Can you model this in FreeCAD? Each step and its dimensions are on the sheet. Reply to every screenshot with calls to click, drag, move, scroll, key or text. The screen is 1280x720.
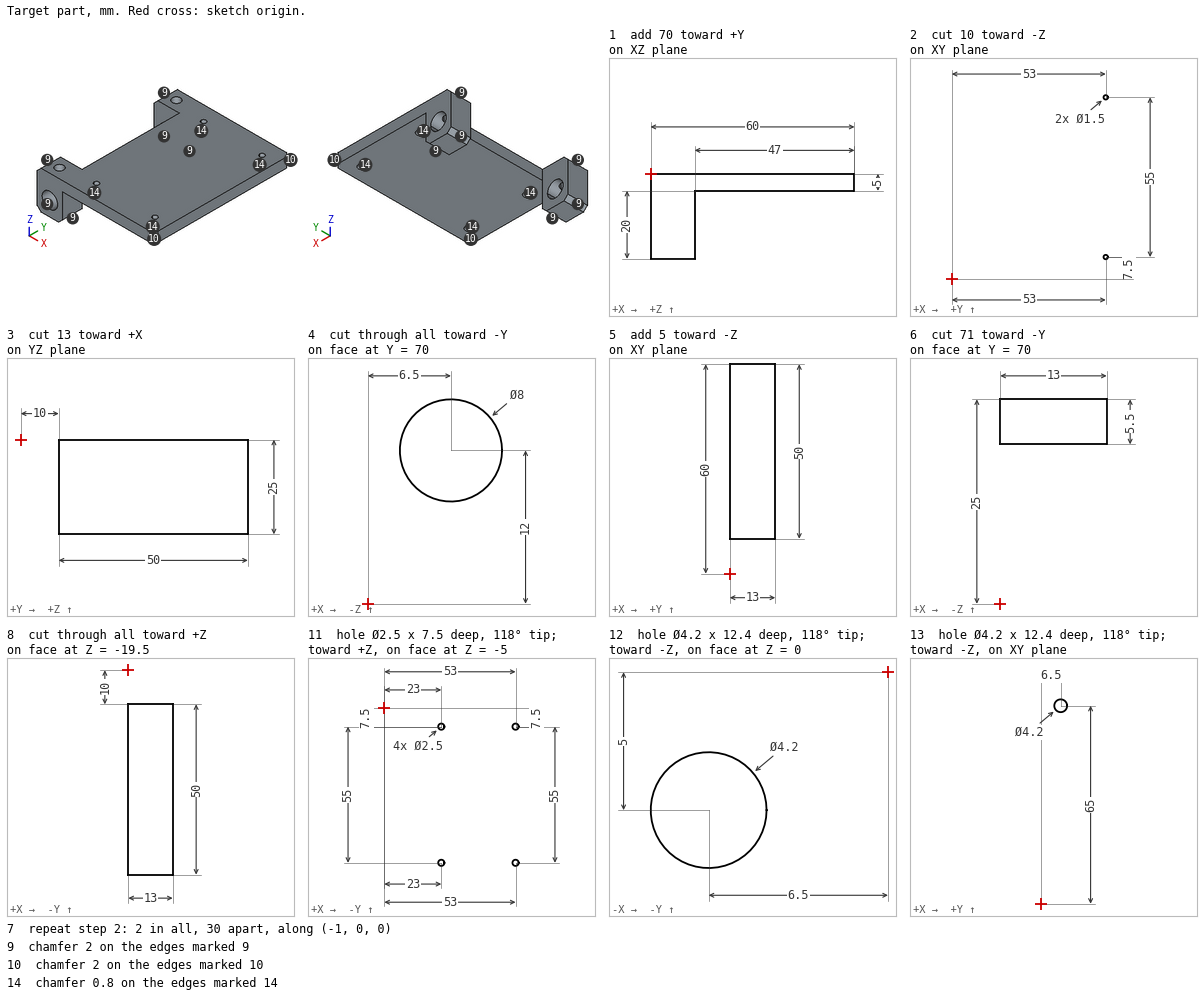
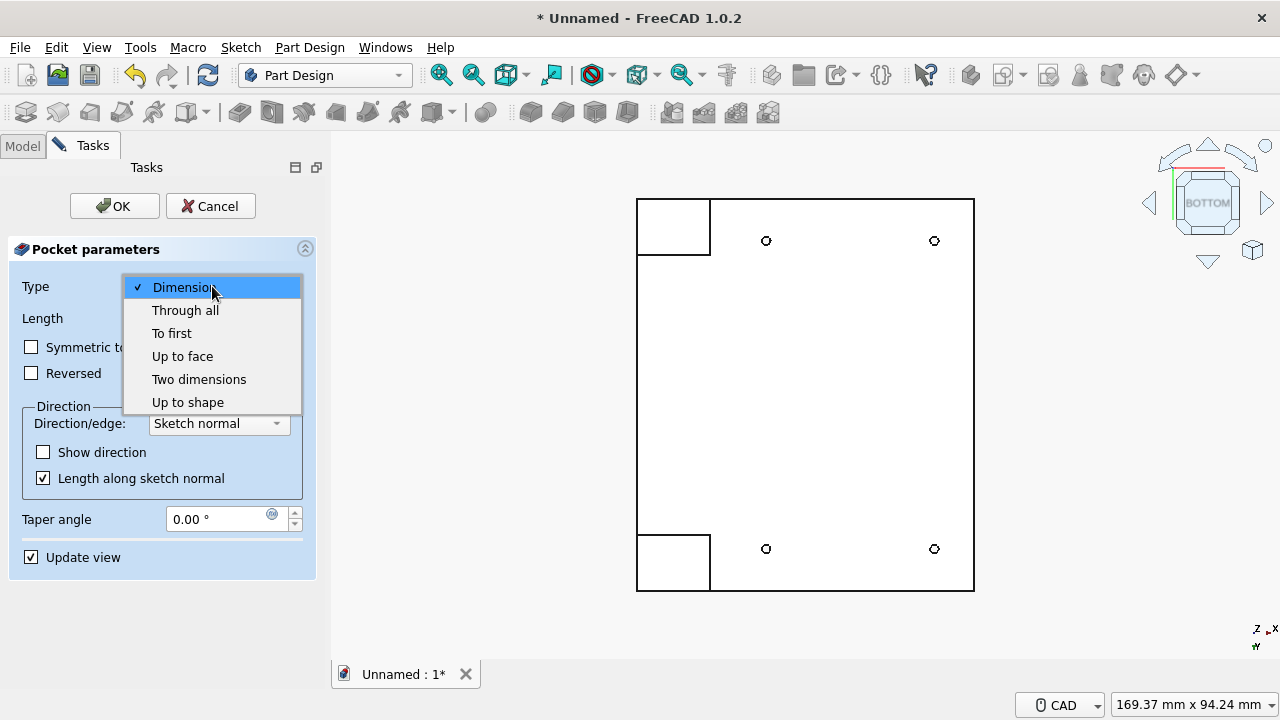
click(212, 310)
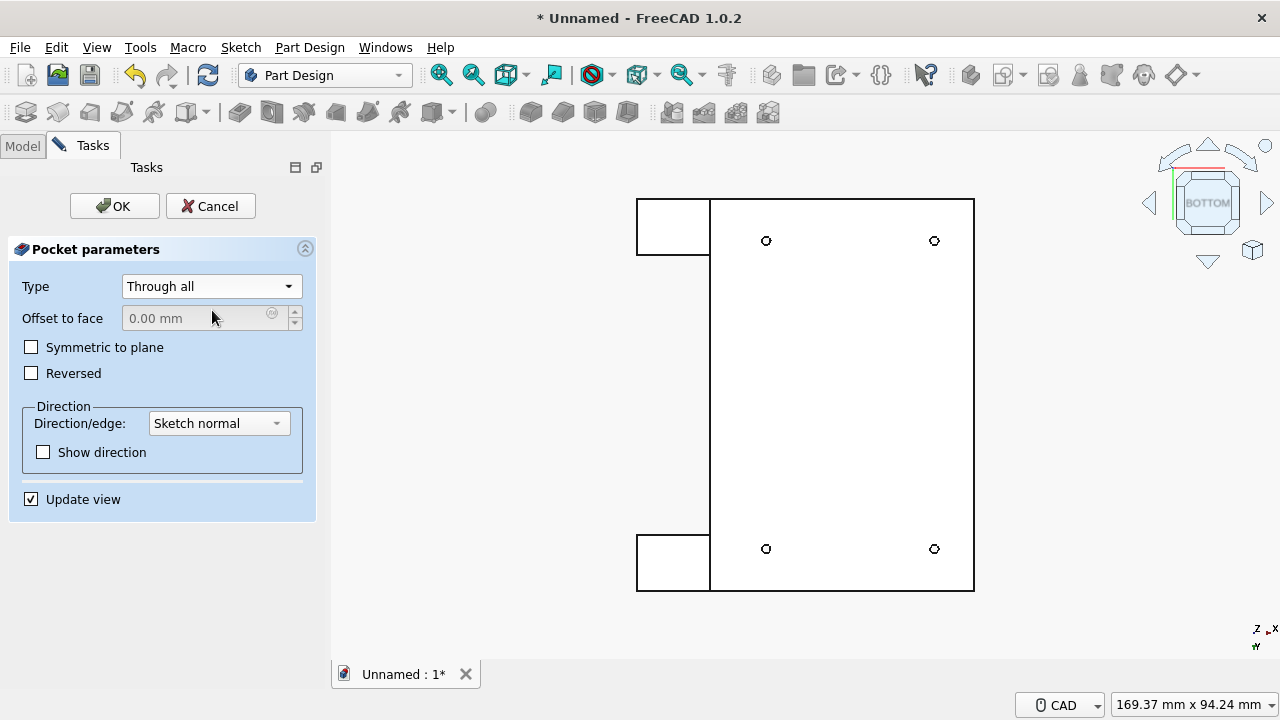
click(115, 206)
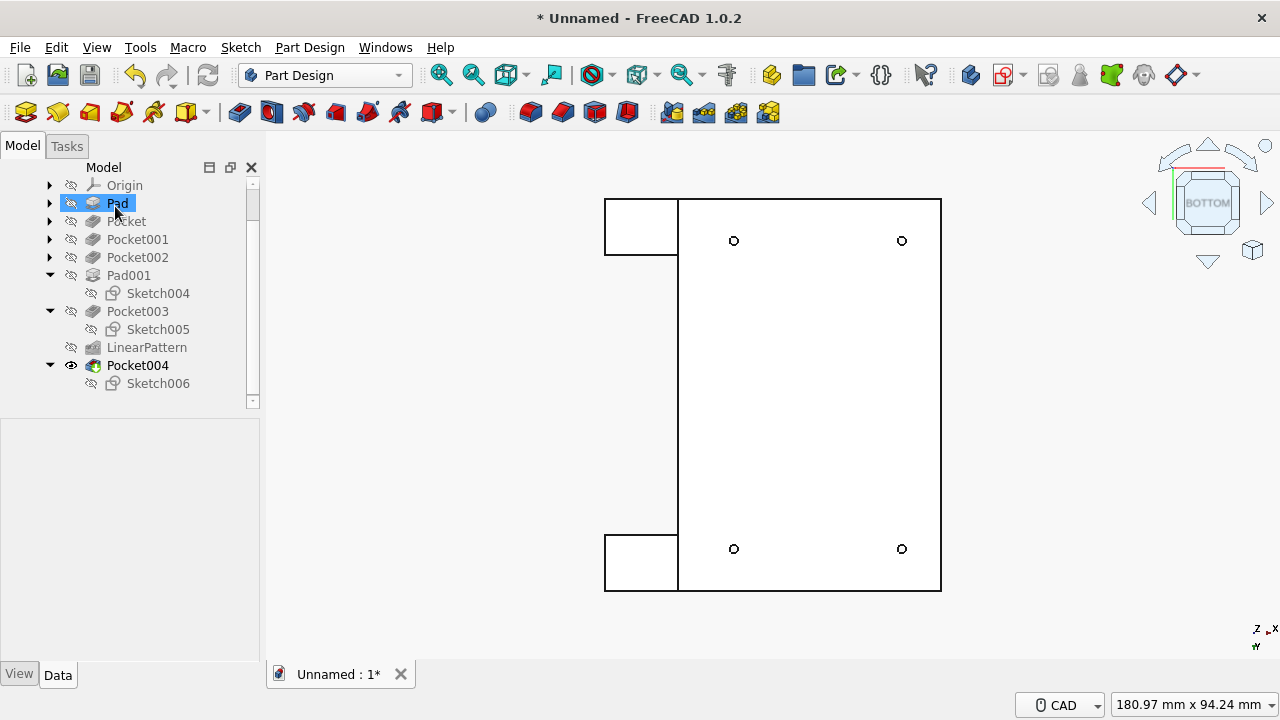
click(605, 226)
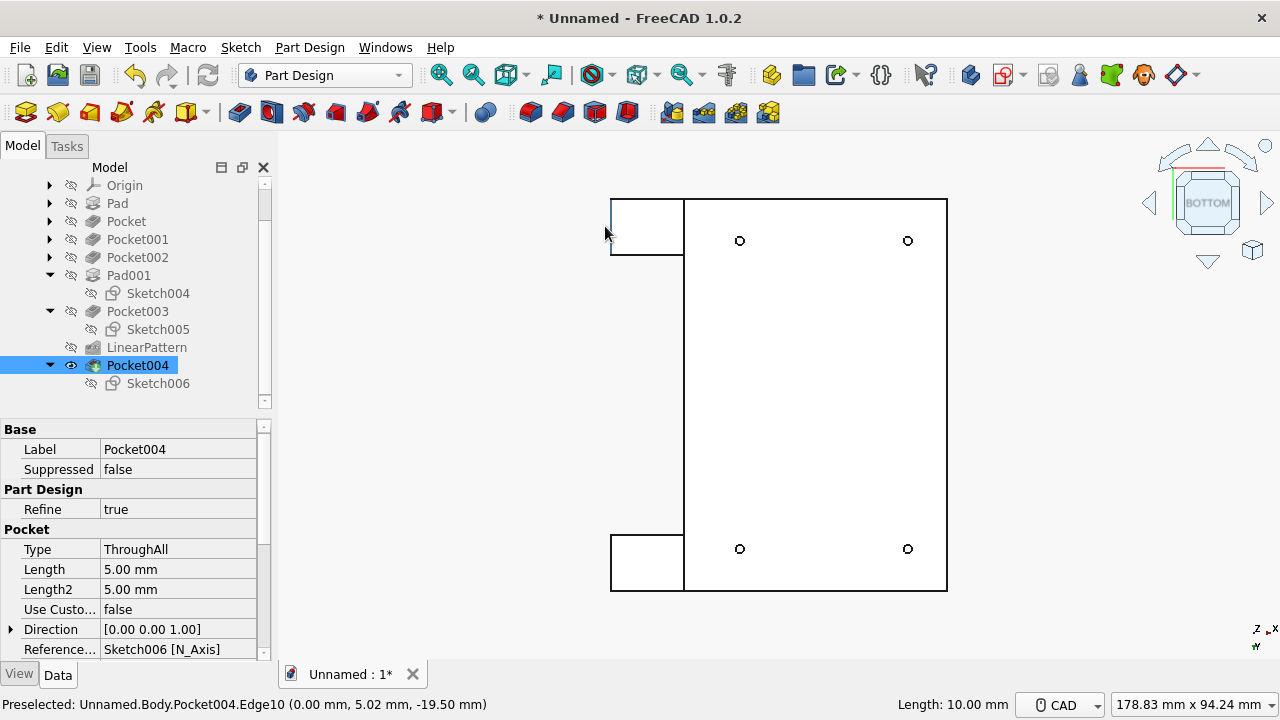
click(611, 562, ctrl)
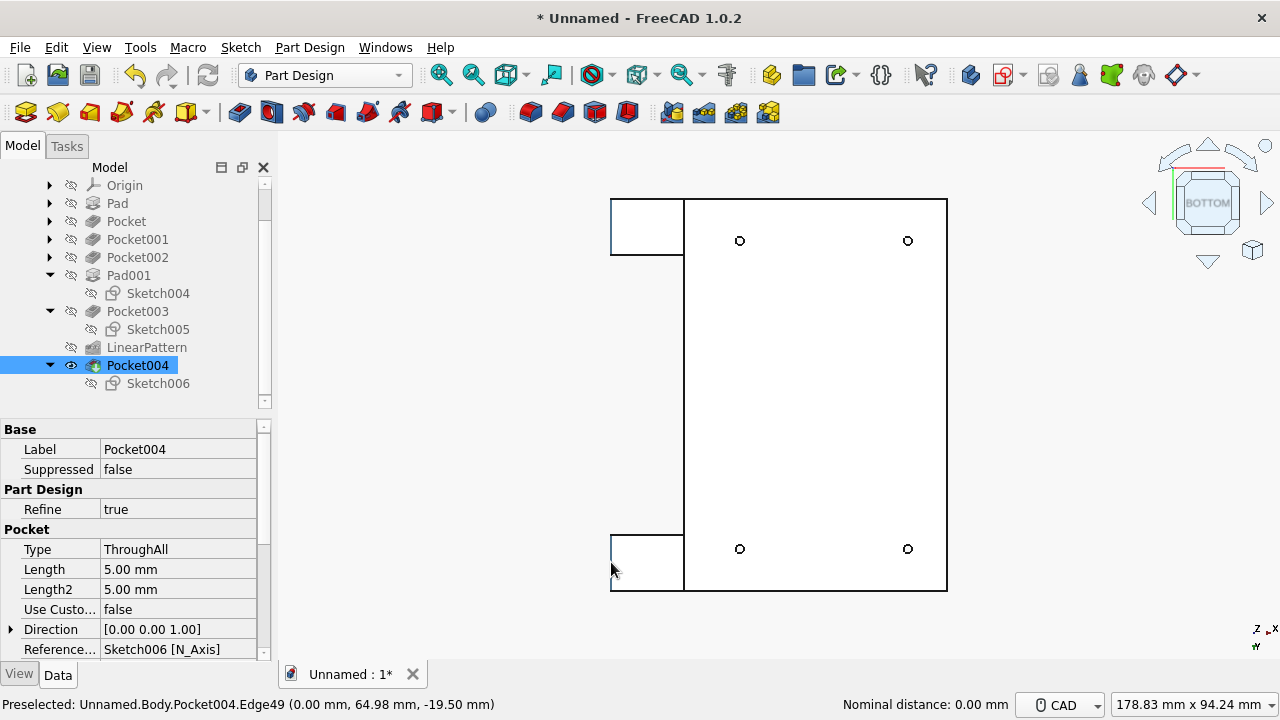
click(684, 226, ctrl)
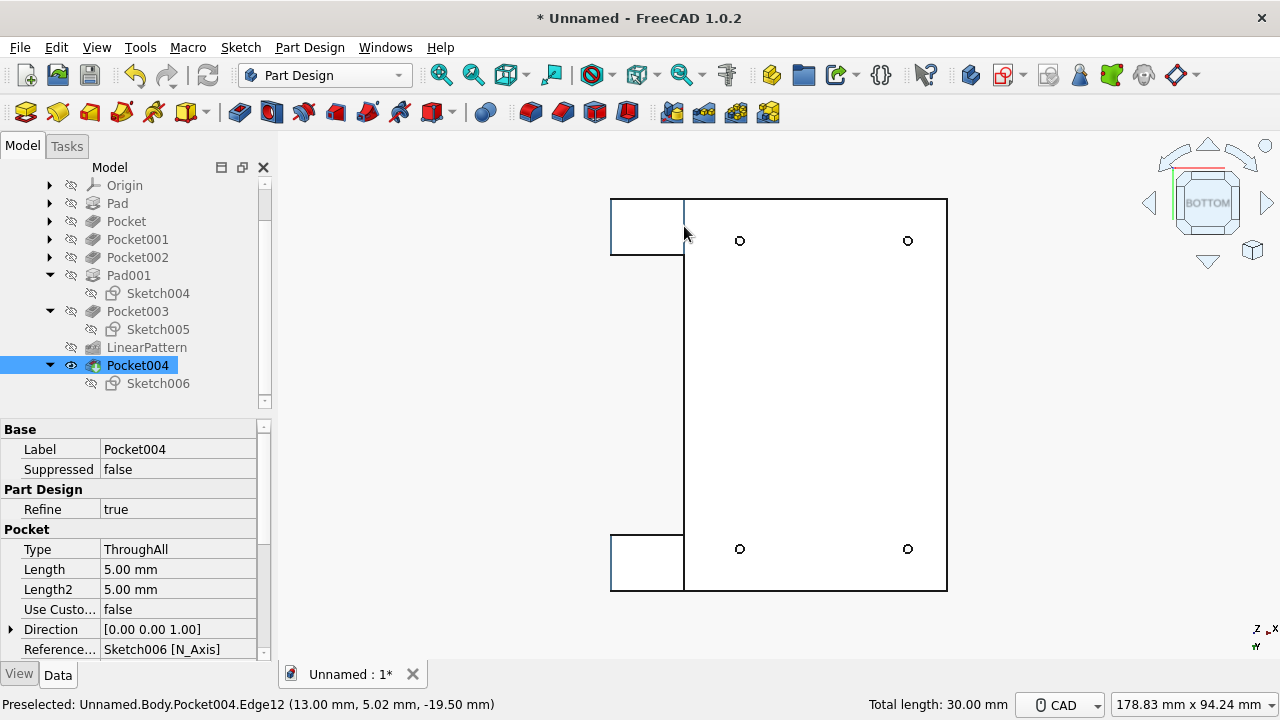
click(684, 562, ctrl)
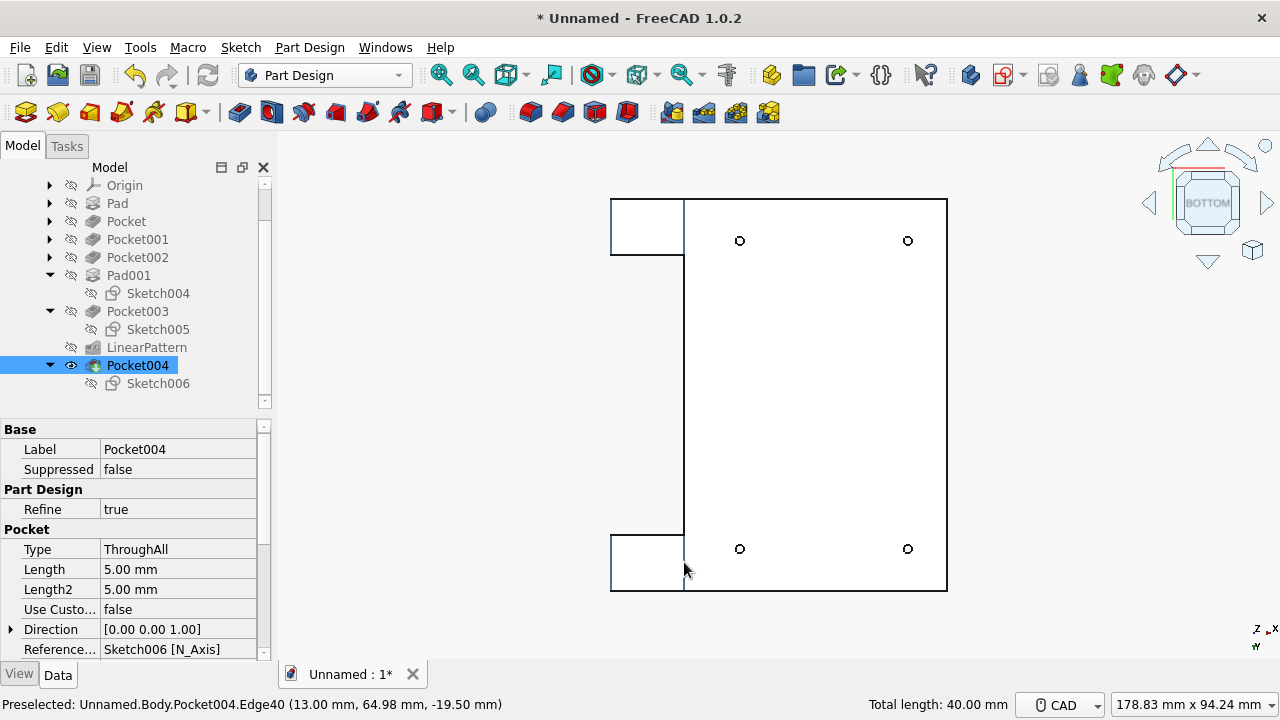
key(0)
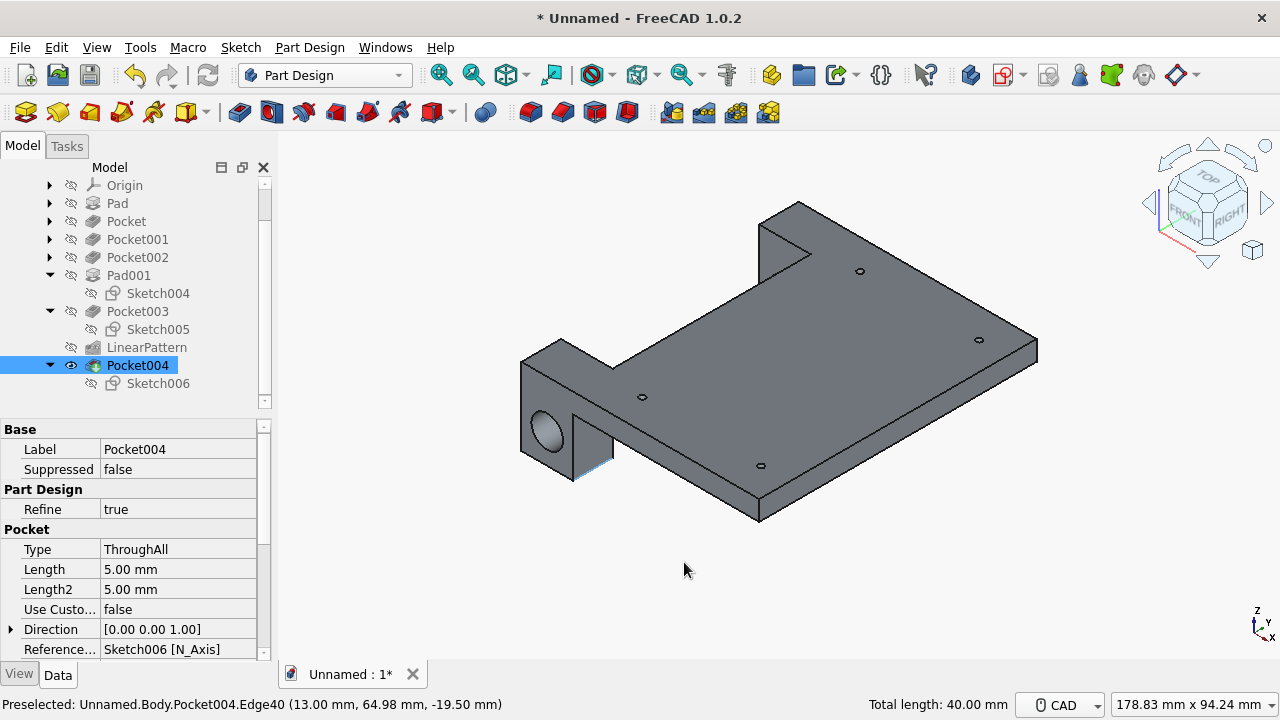
key(2)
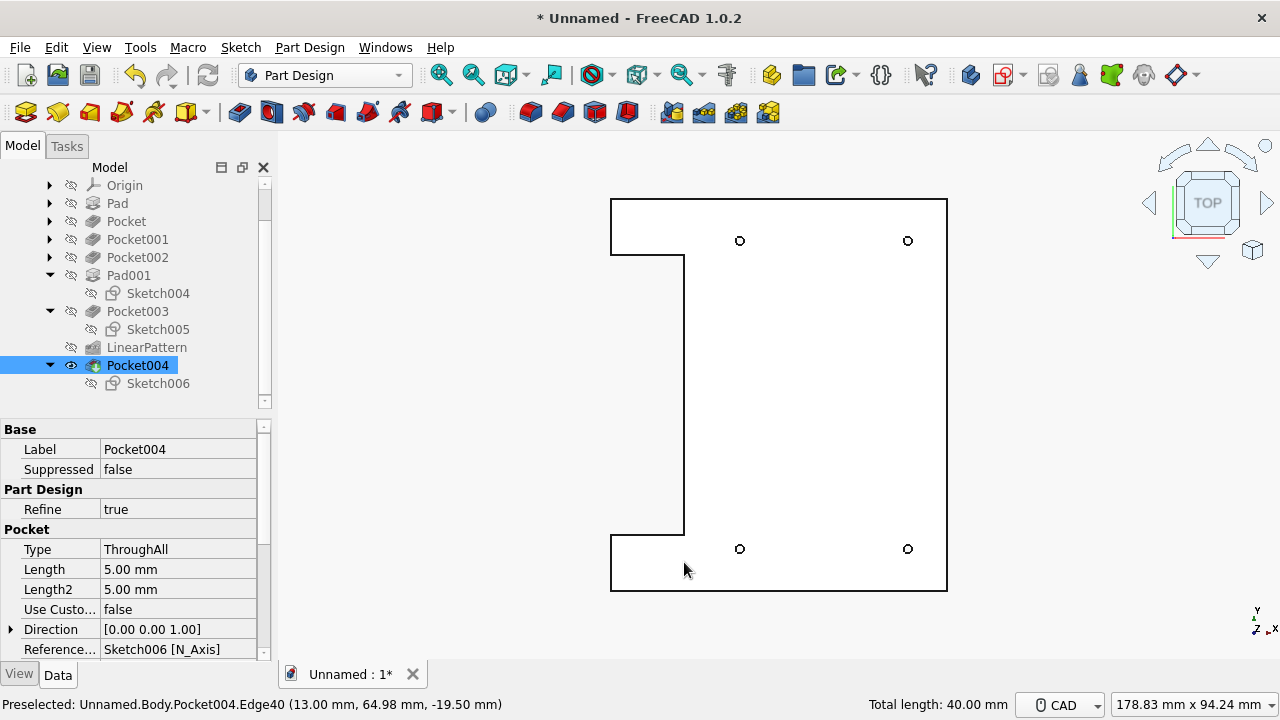
key(1)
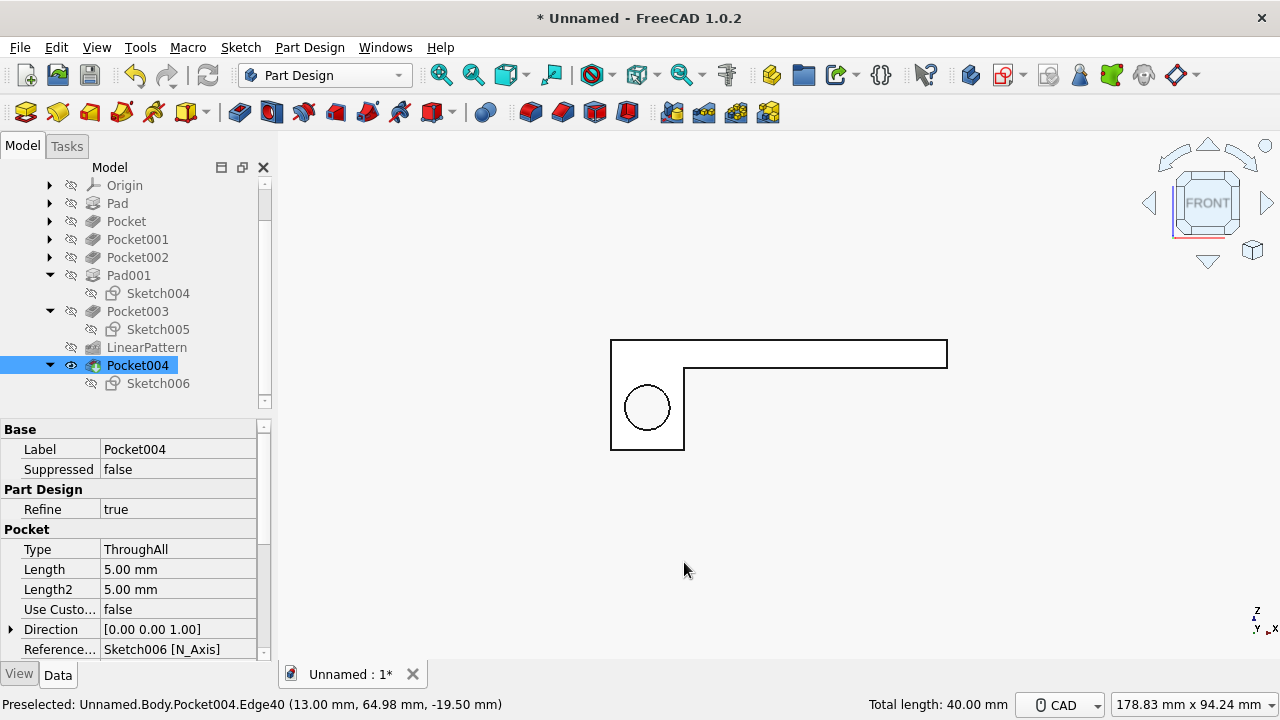
click(442, 76)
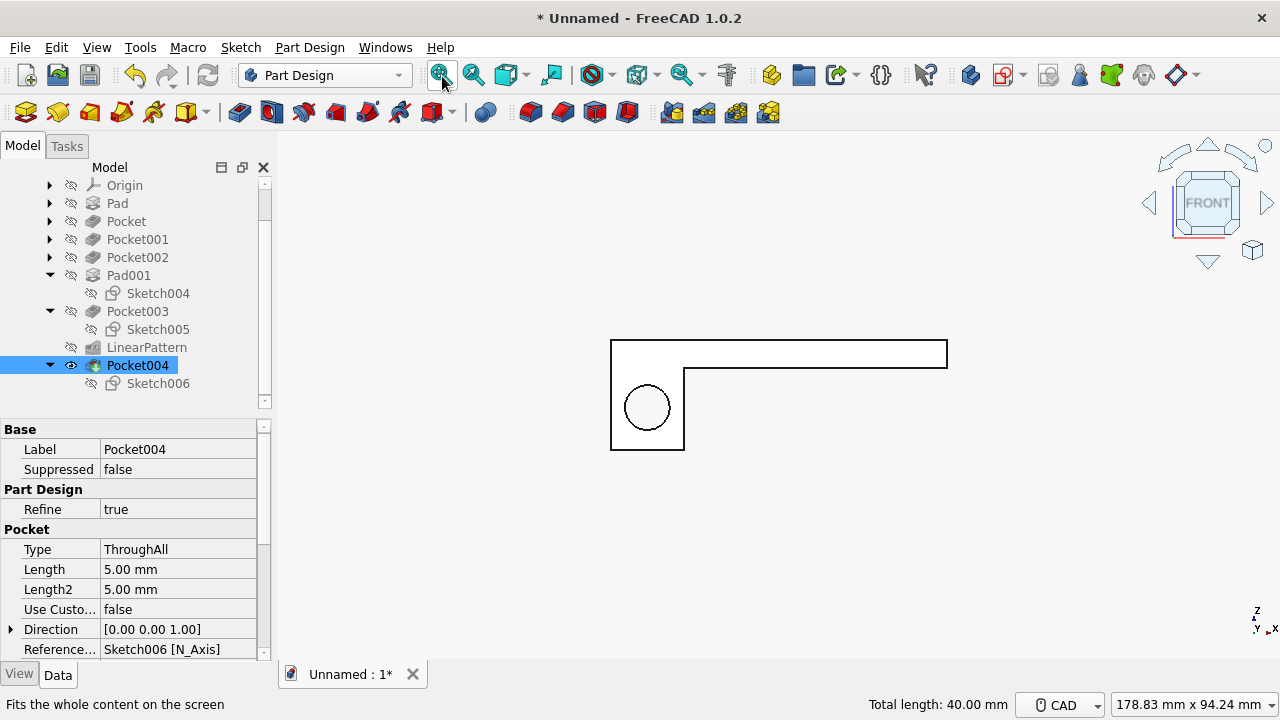
key(3)